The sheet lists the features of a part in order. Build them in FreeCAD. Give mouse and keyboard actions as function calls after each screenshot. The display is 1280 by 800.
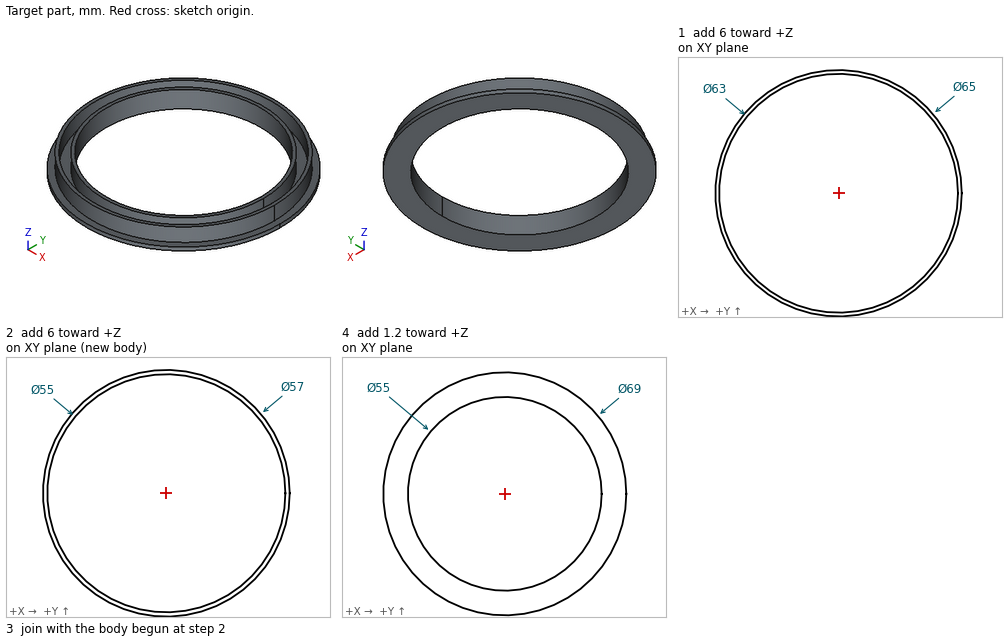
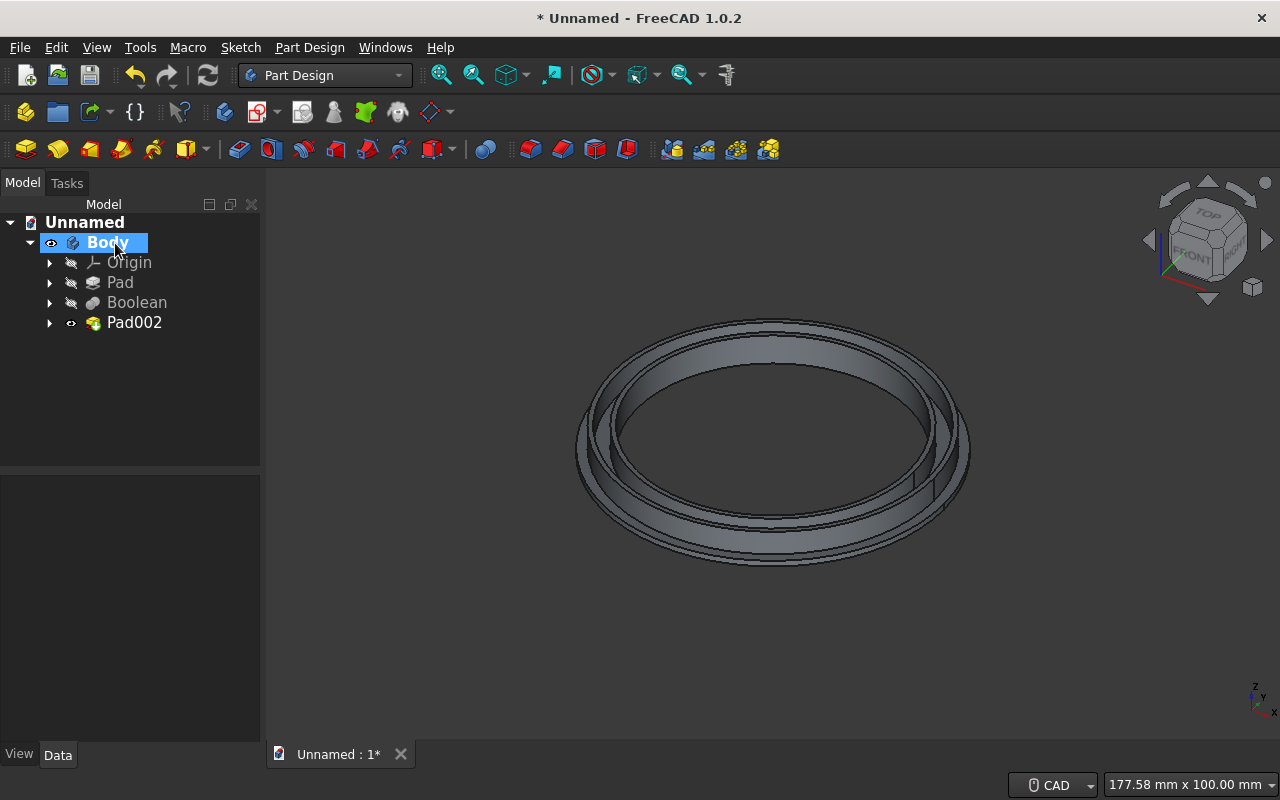
key(0)